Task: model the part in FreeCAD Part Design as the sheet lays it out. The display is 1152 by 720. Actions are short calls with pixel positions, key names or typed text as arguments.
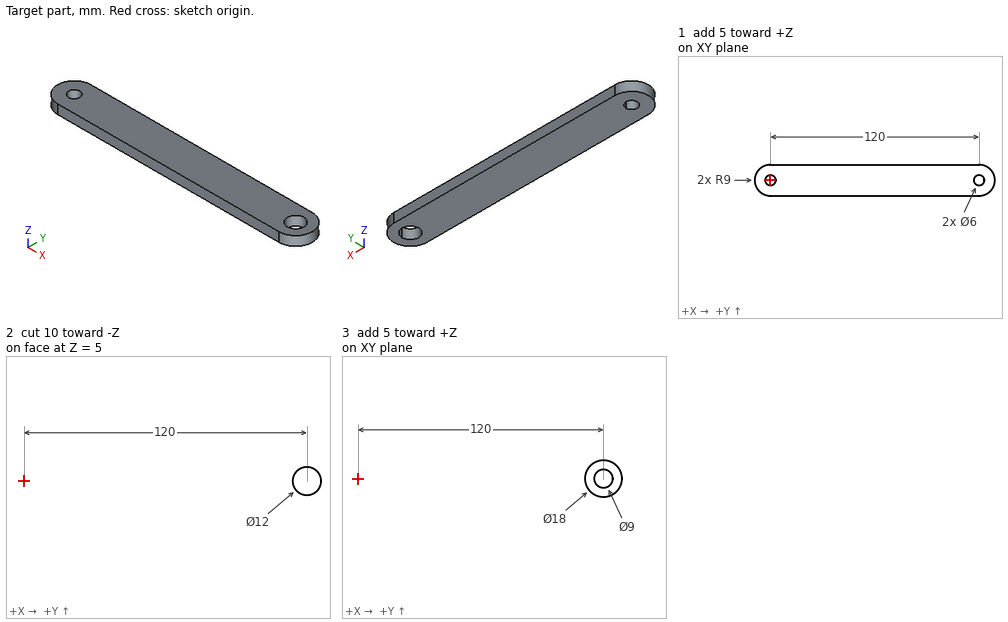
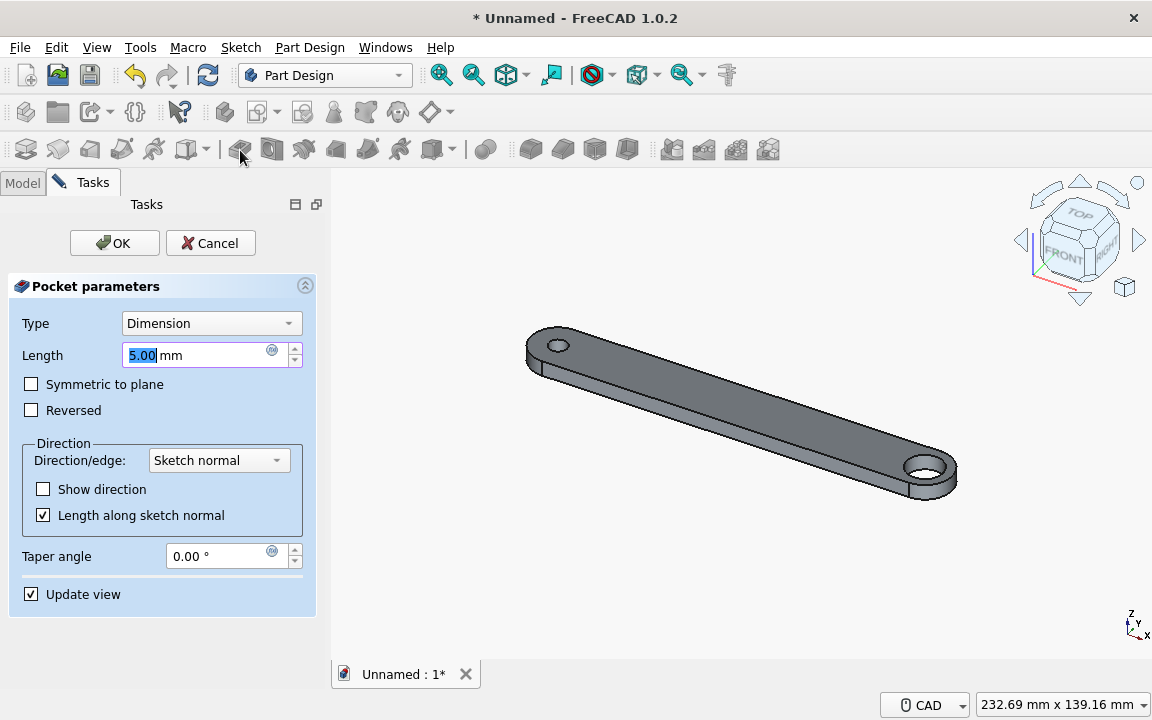
text(10)
key(Tab)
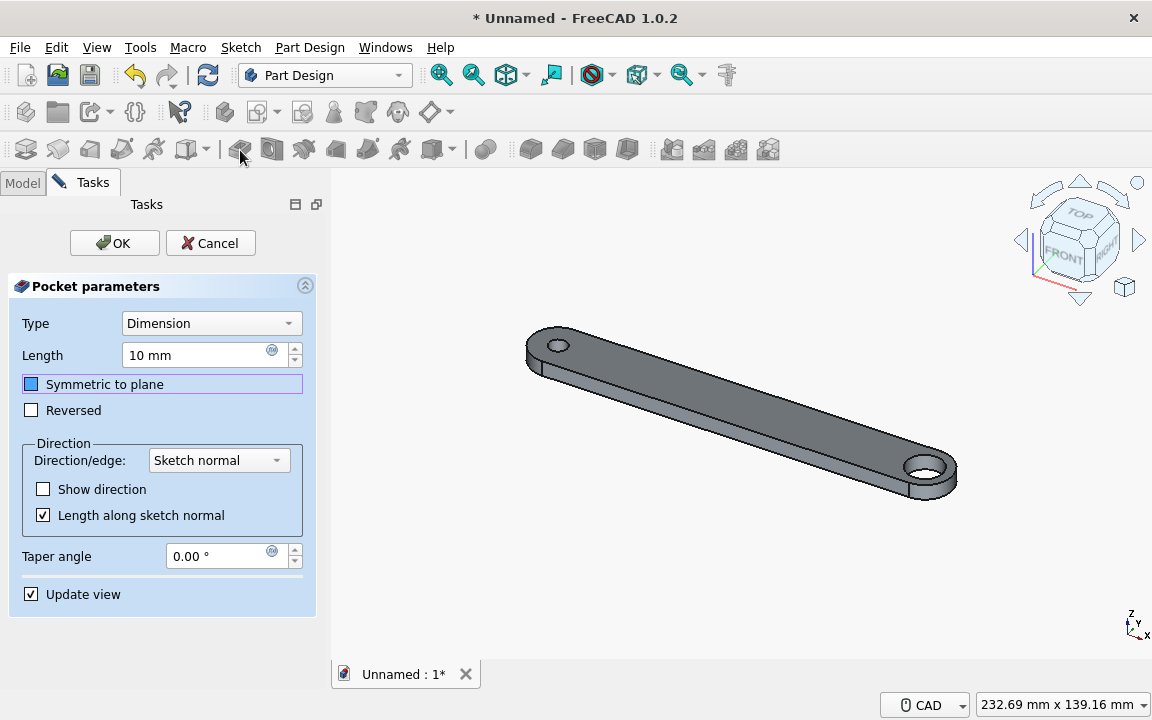
click(115, 243)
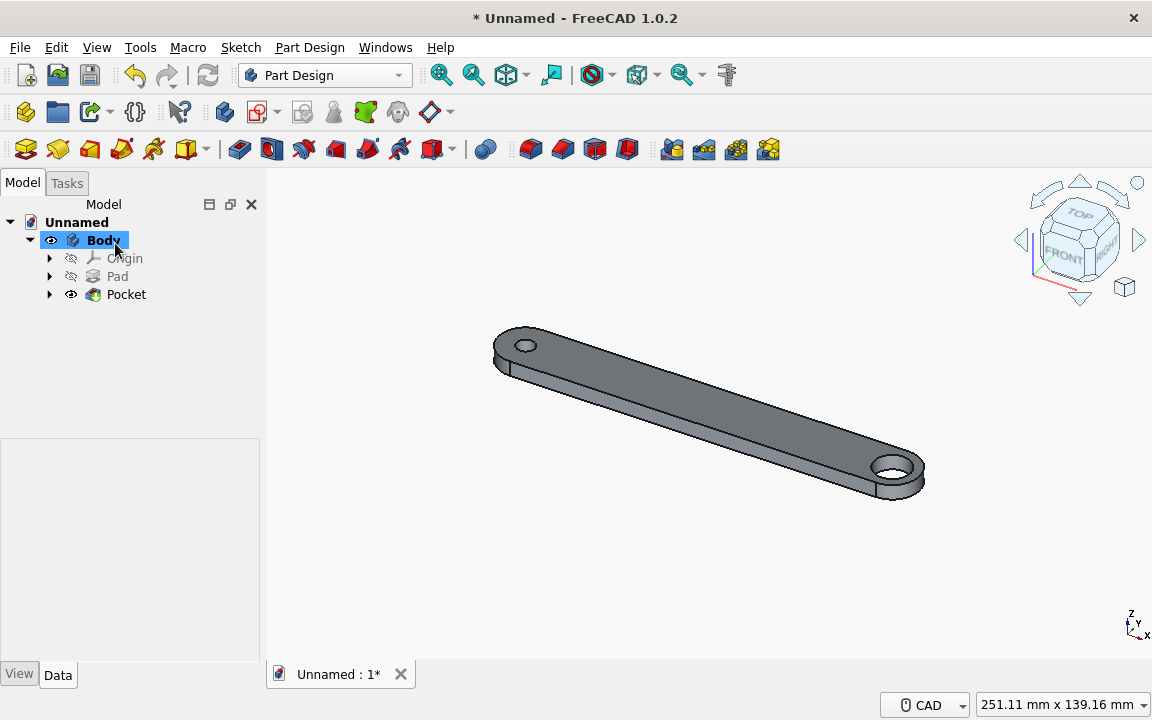
click(258, 112)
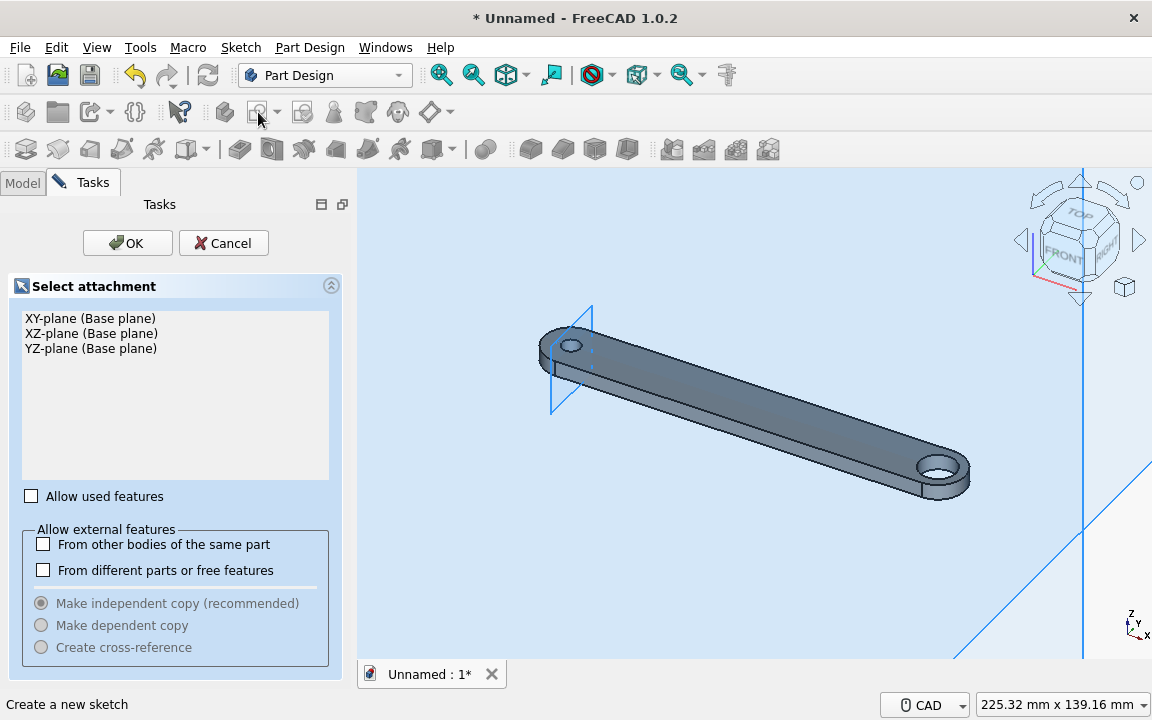
click(82, 318)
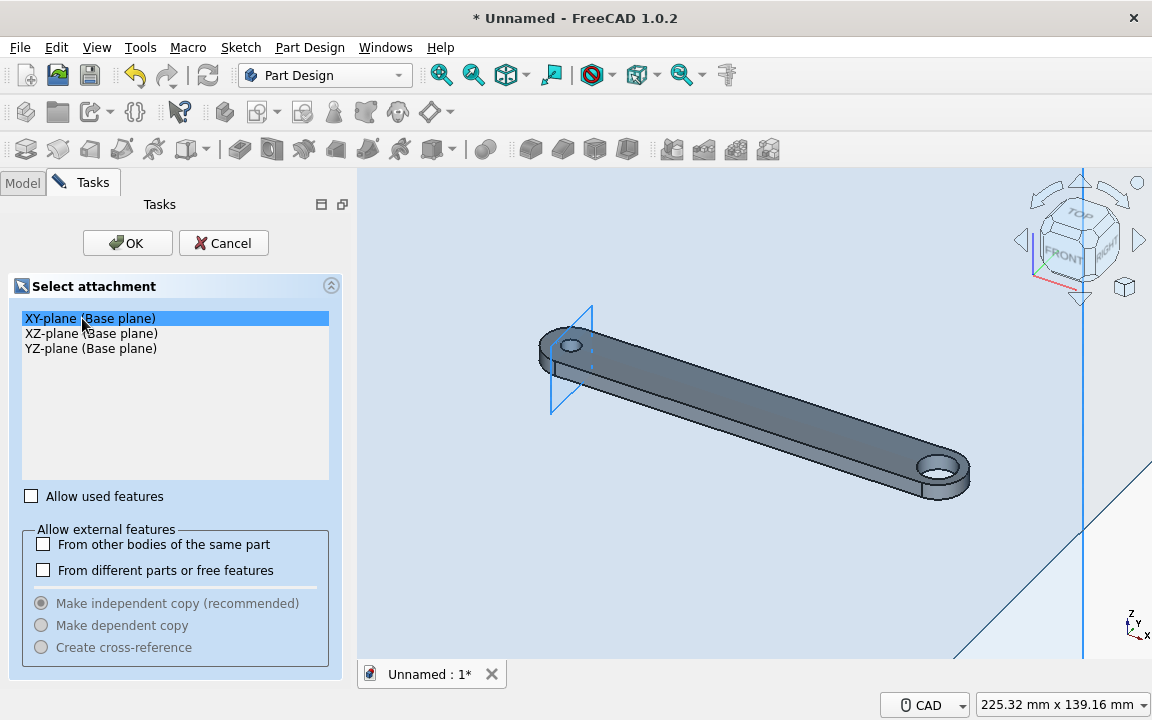
click(128, 243)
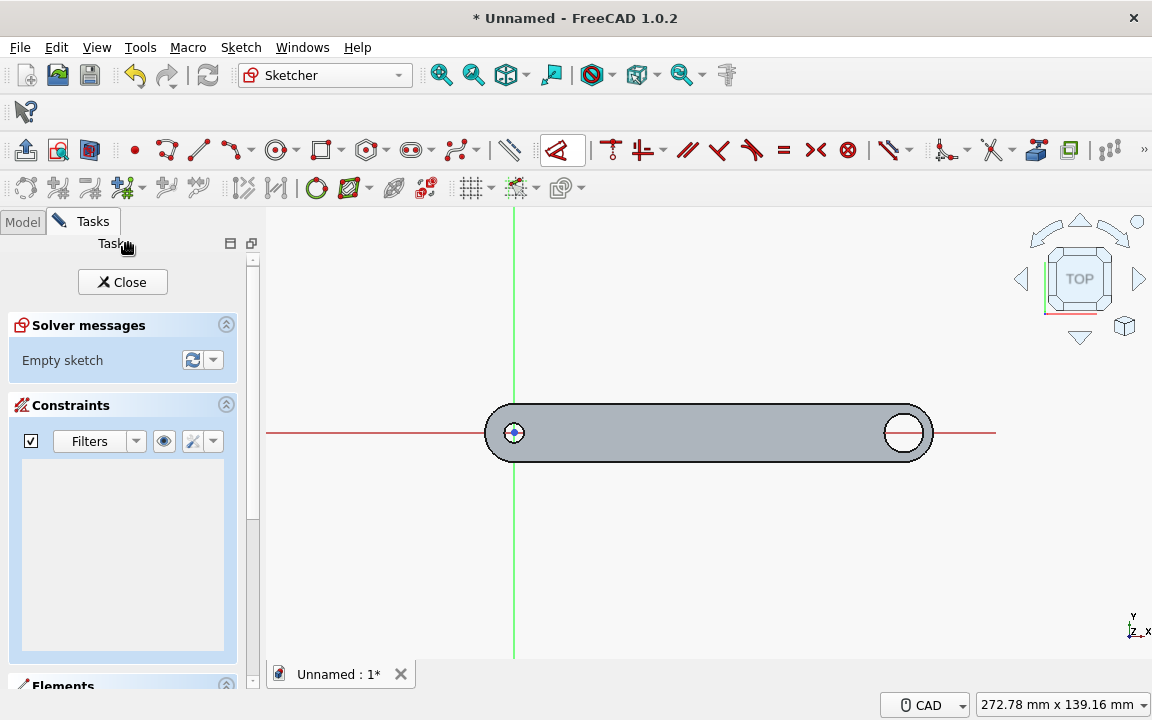
click(90, 150)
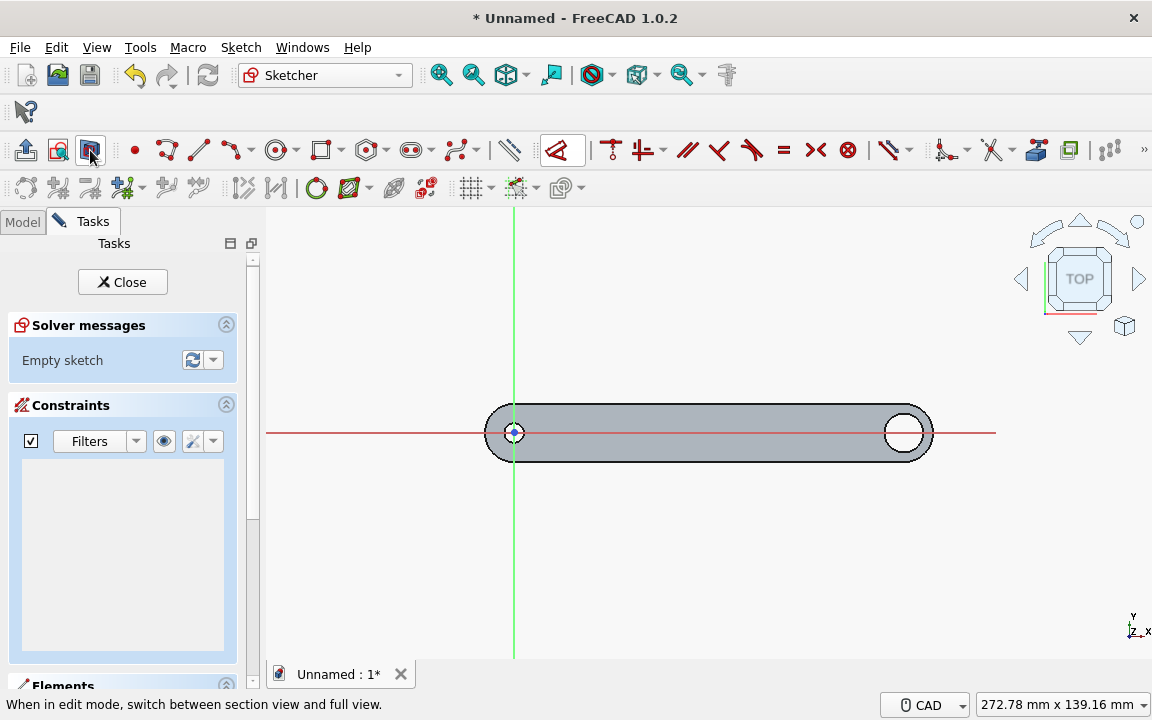
scroll(971, 433, up, 8)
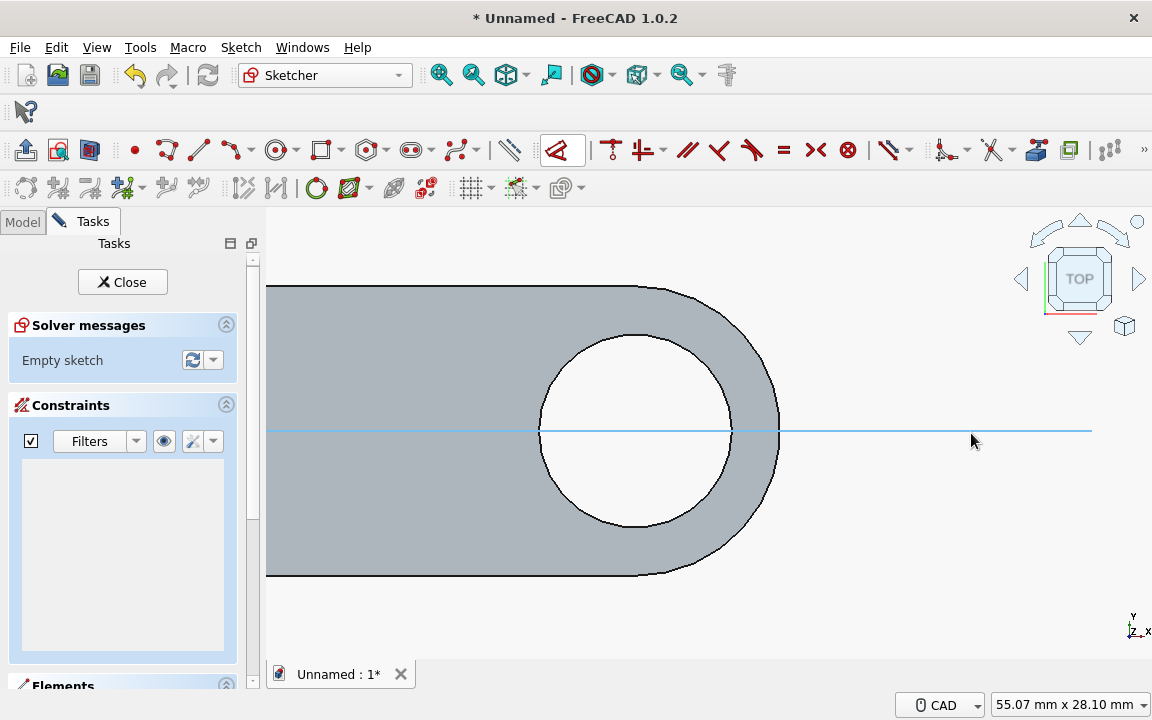
click(276, 150)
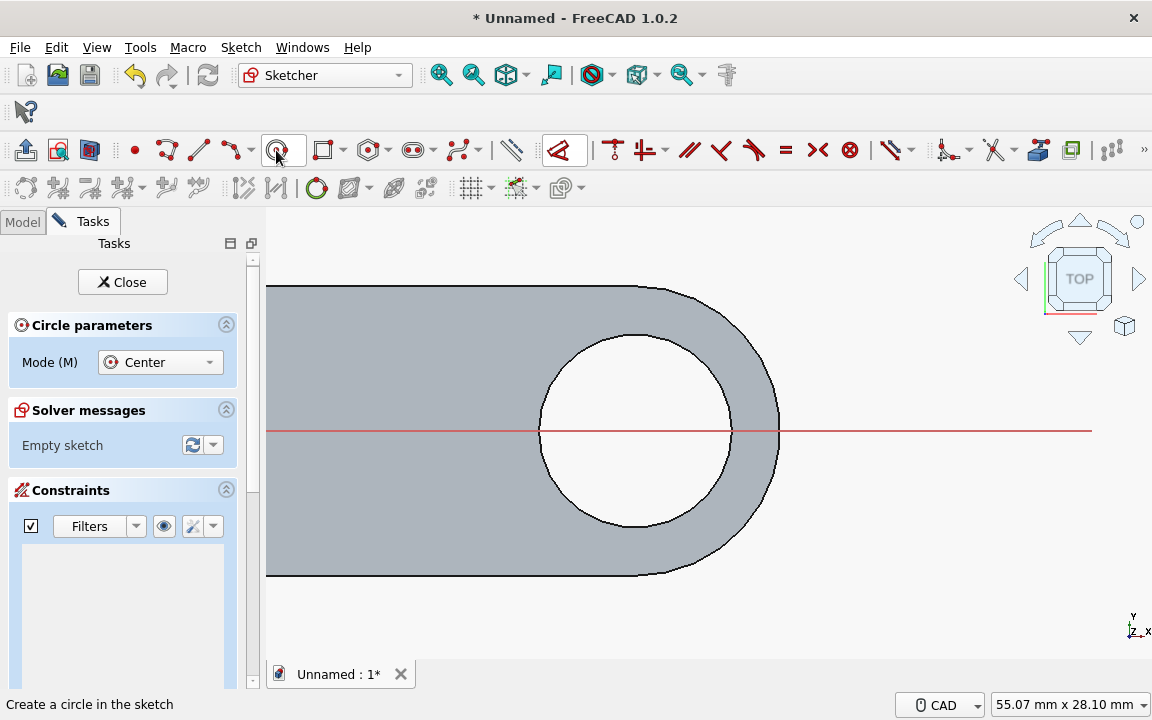
click(635, 431)
move(738, 329)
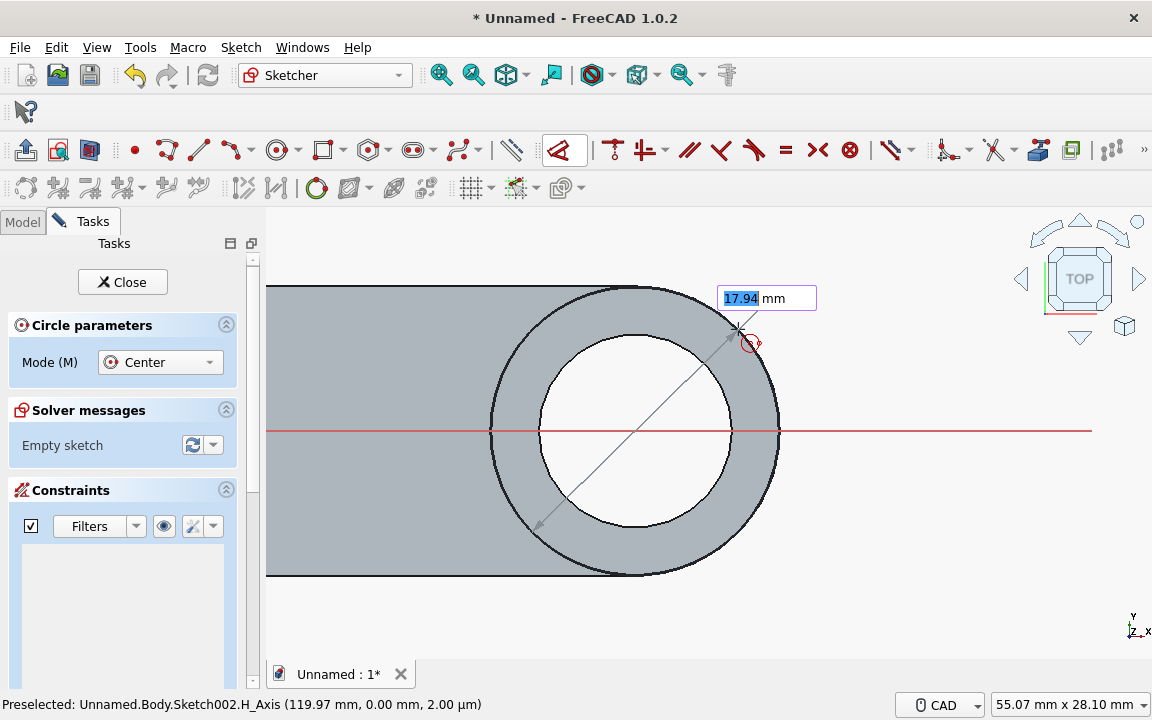
text(18)
key(Return)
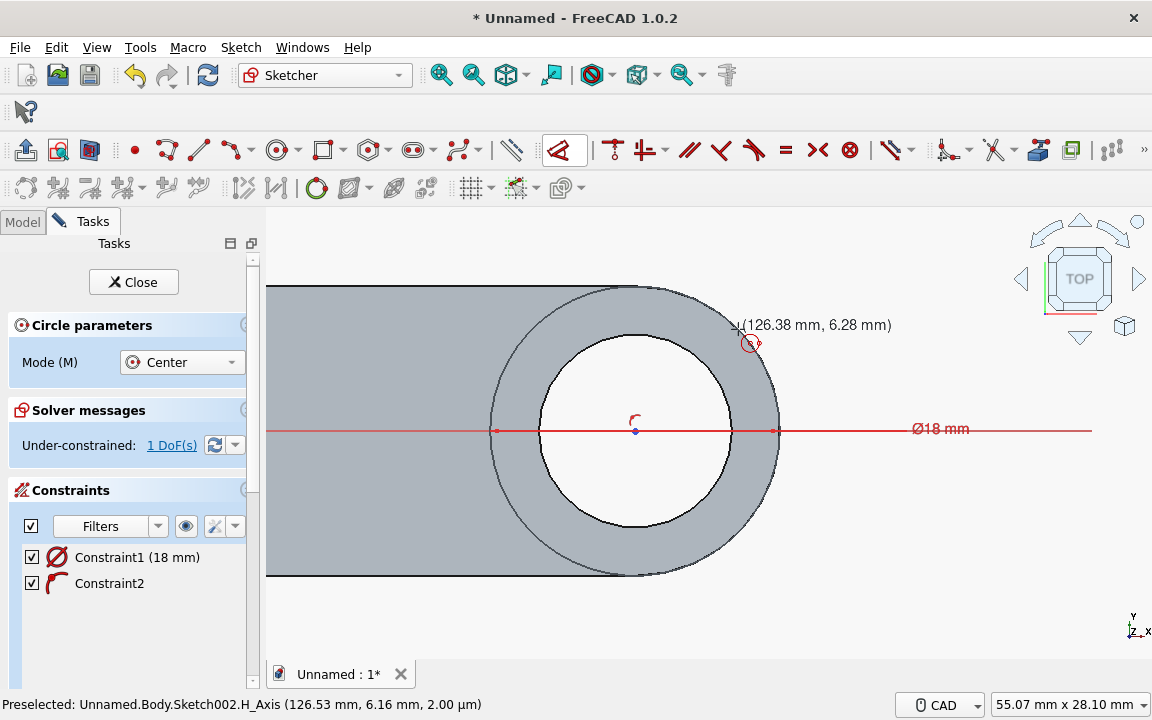
click(635, 431)
move(687, 380)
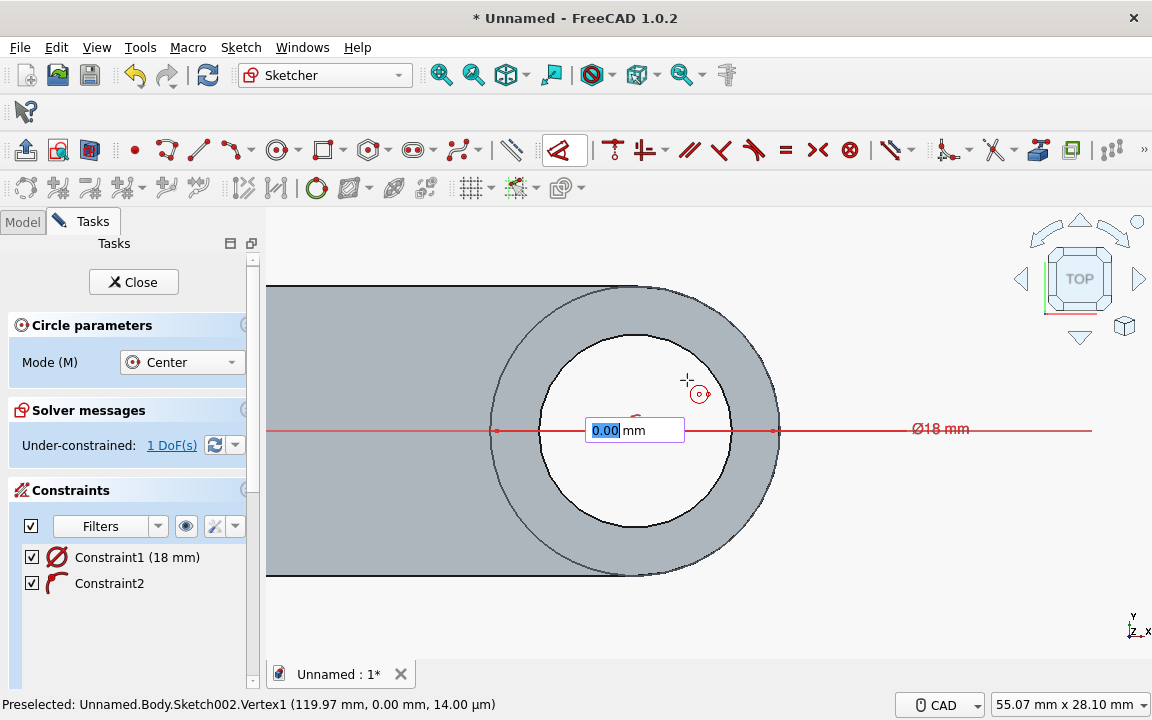
text(9)
key(Return)
key(Escape)